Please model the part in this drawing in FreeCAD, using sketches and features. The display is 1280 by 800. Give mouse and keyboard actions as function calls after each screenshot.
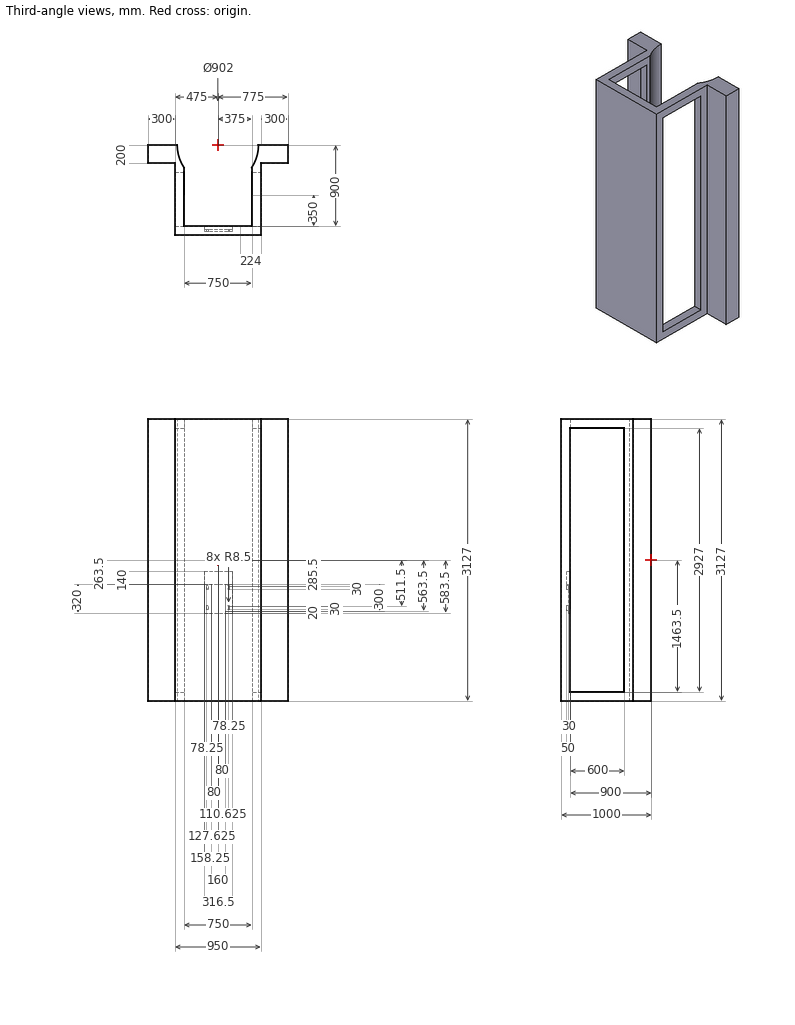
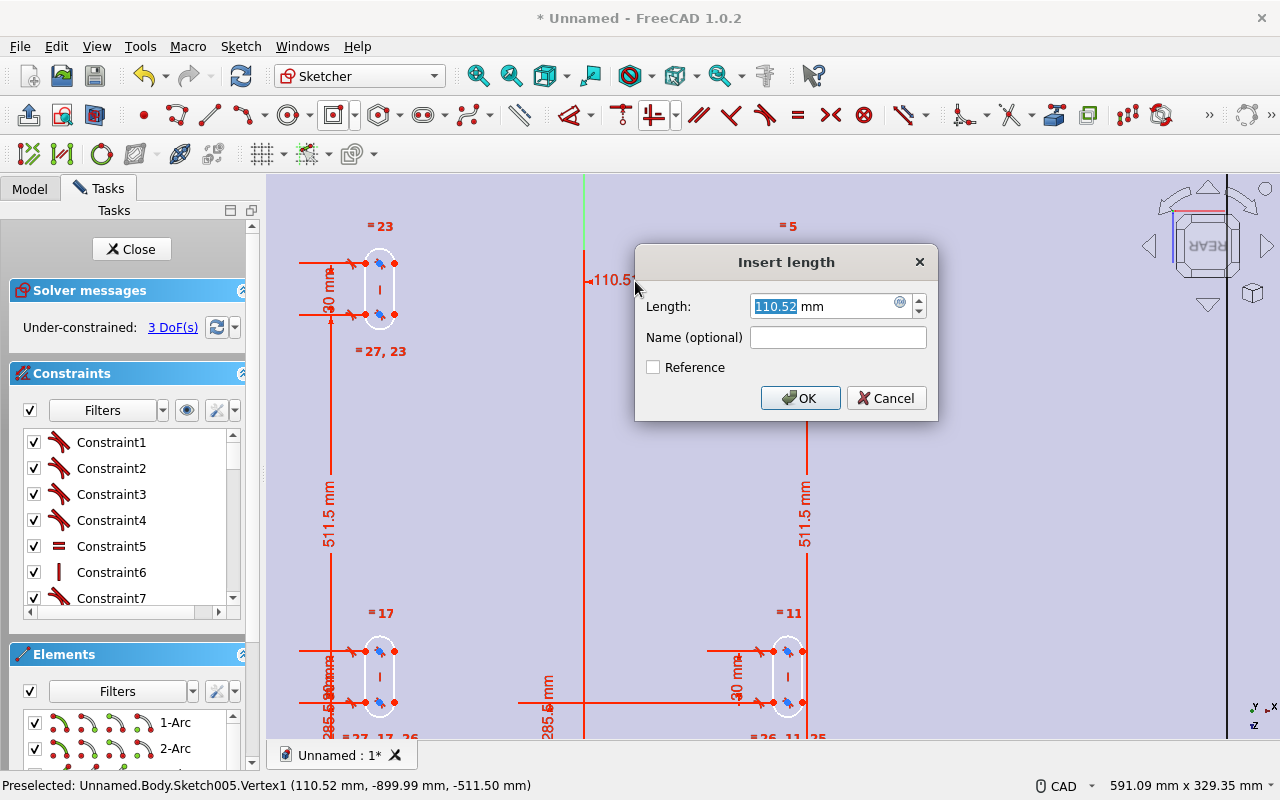
text(110.625)
key(Return)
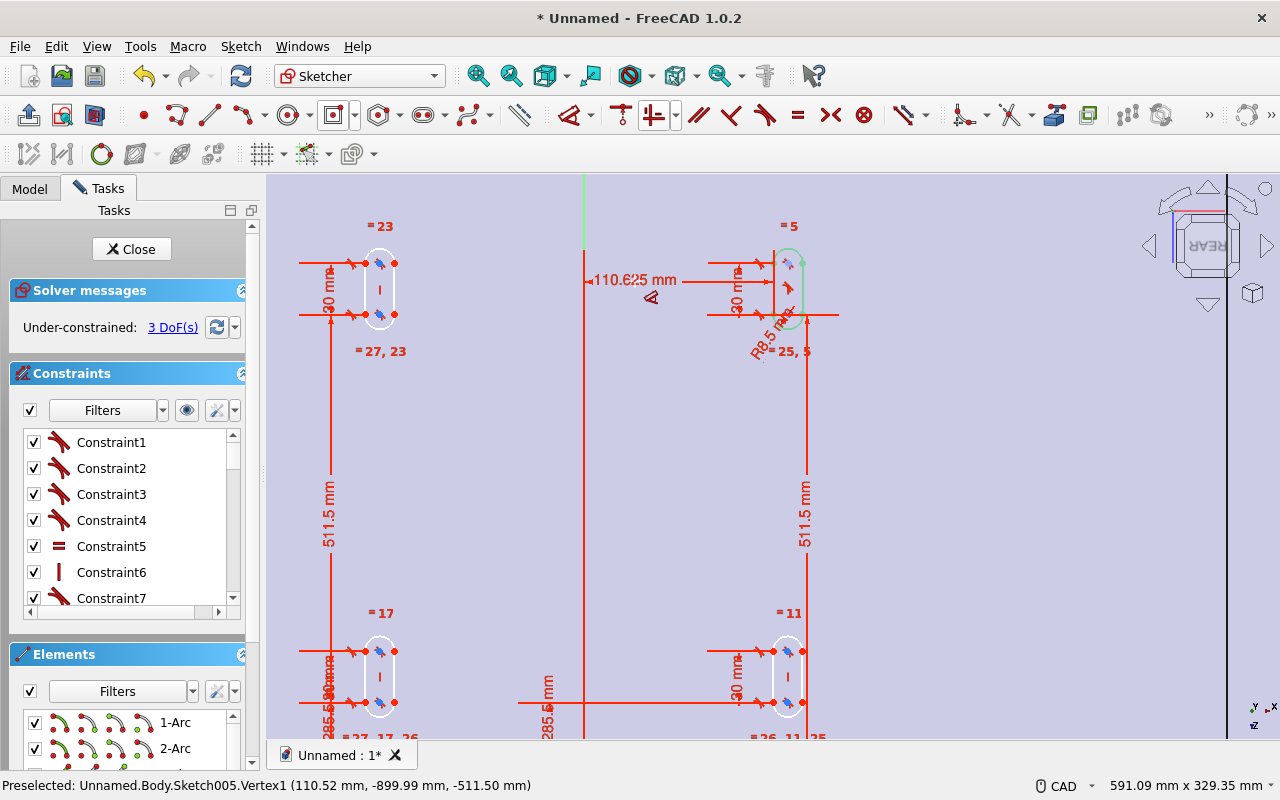
click(773, 703)
click(635, 669)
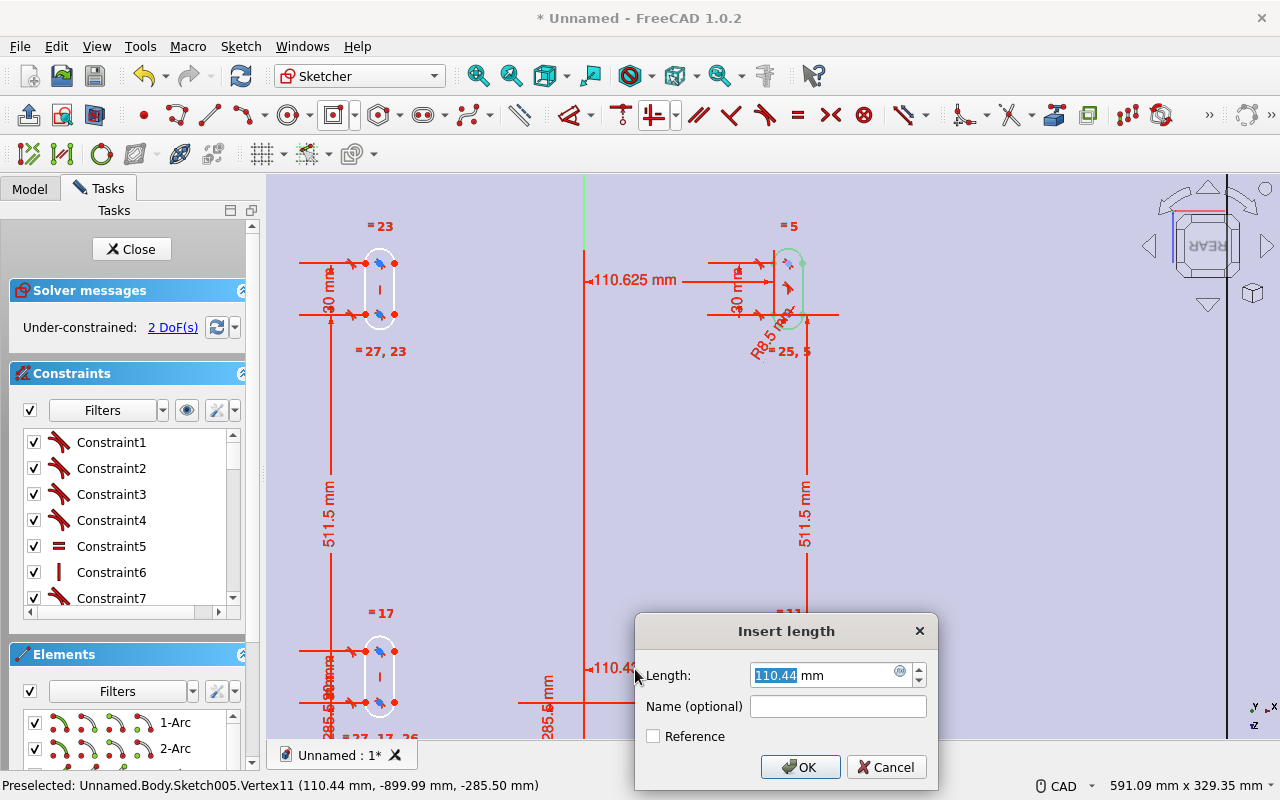
text(110.625)
key(Return)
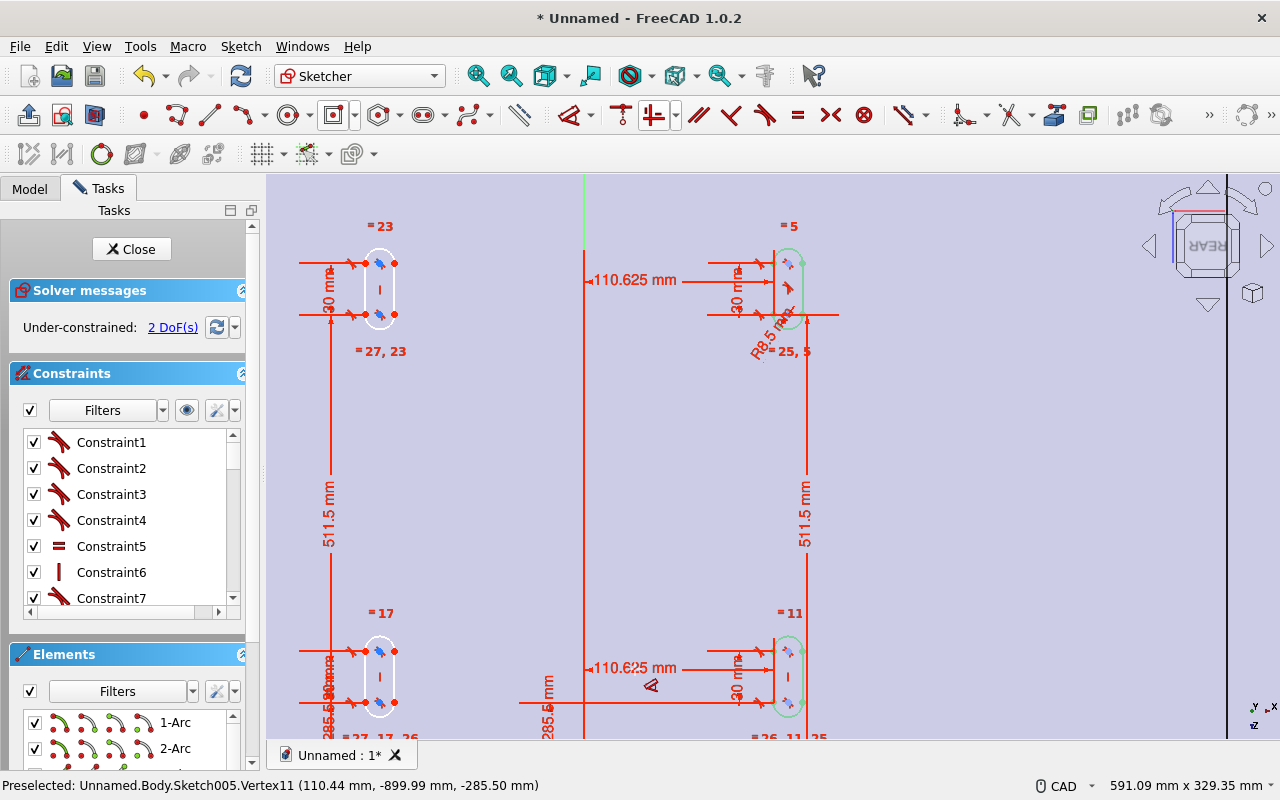
click(365, 703)
click(474, 669)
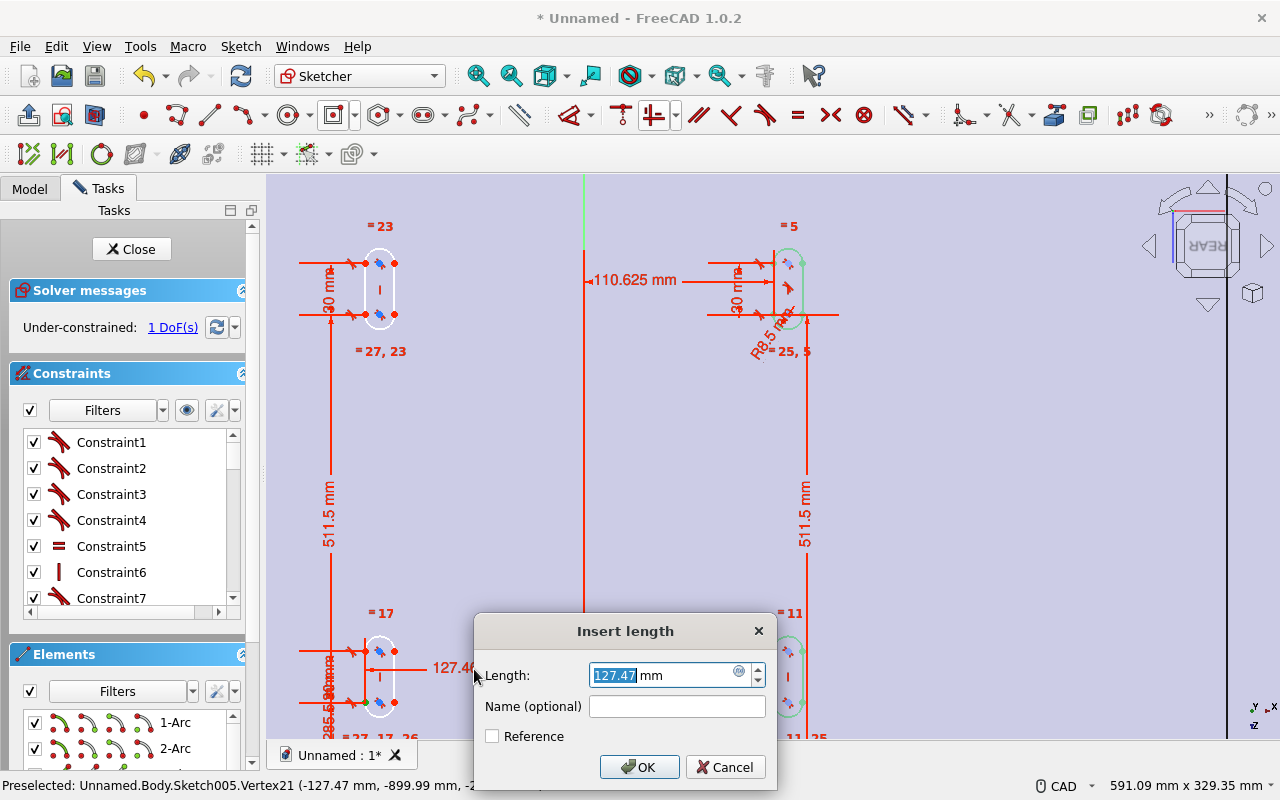
text(127.625)
key(Return)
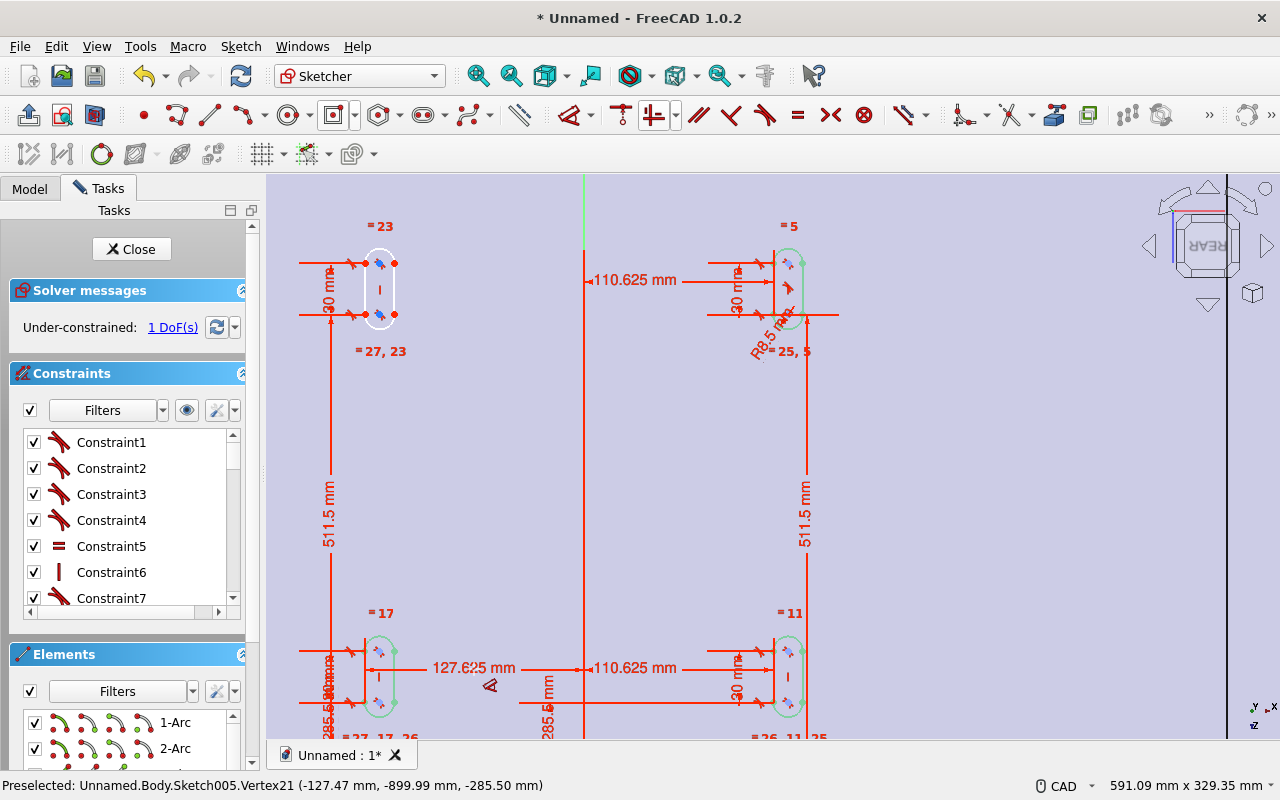
click(365, 315)
click(475, 281)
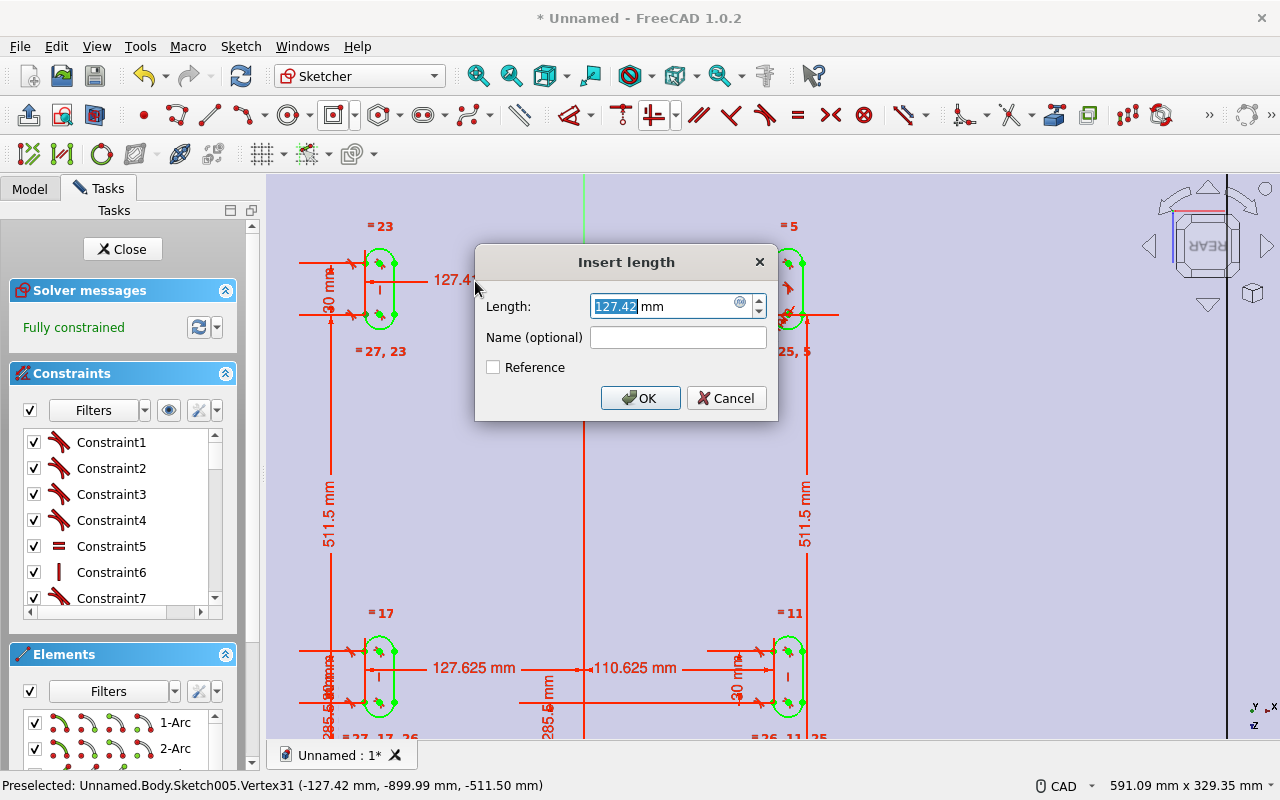
text(127.625)
key(Return)
key(Escape)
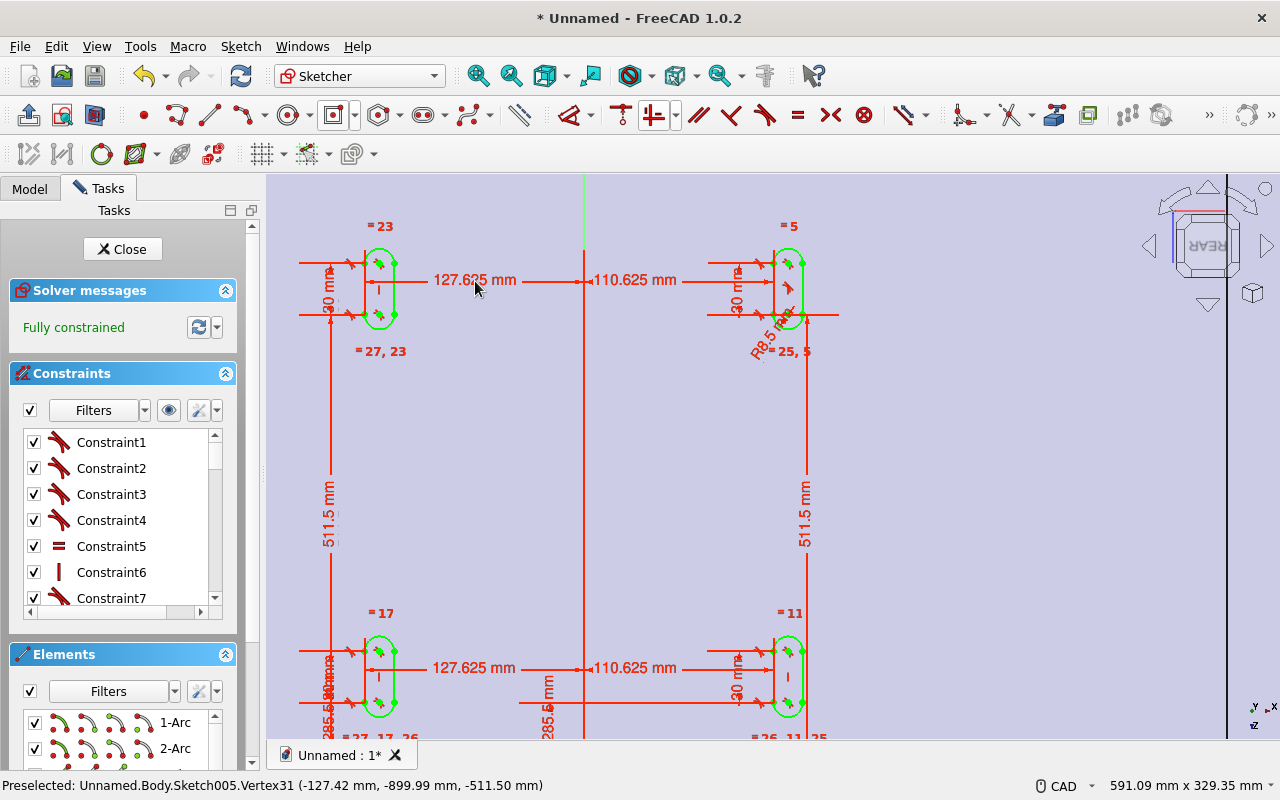
click(123, 249)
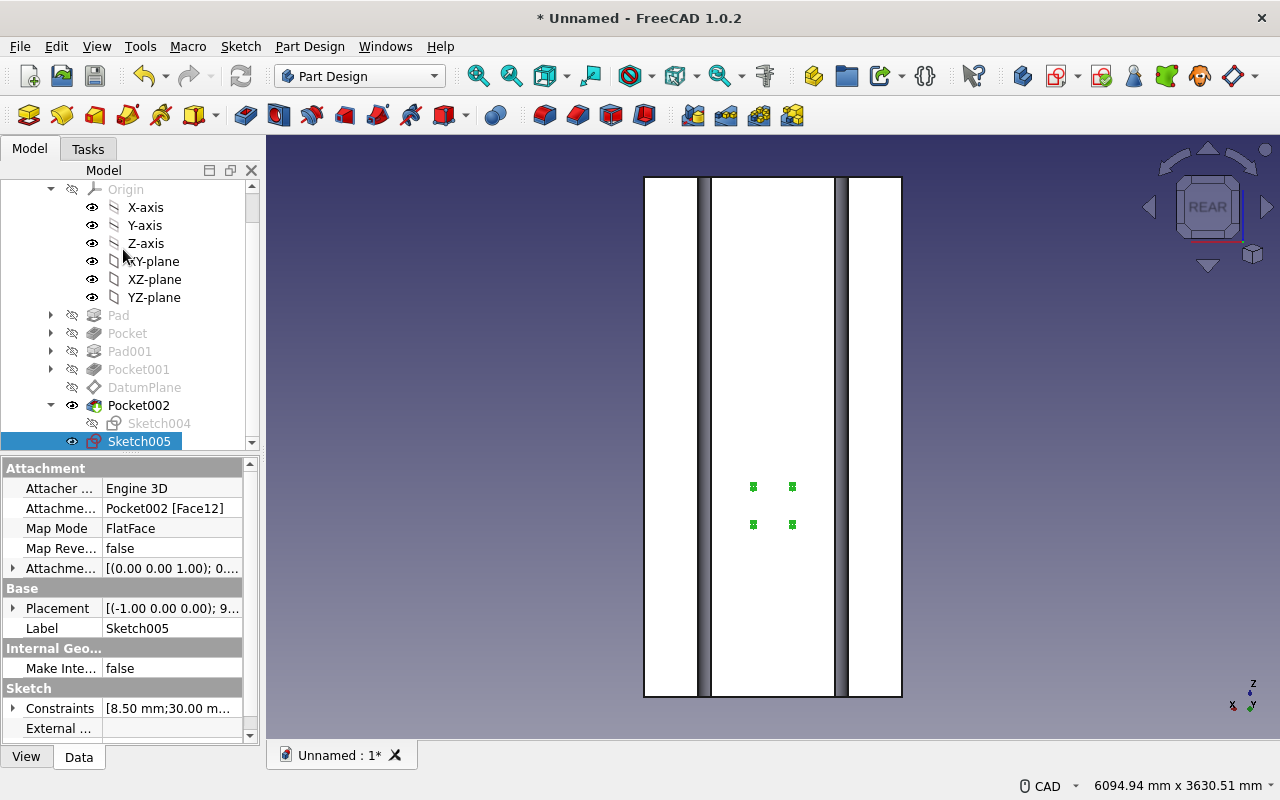
click(246, 116)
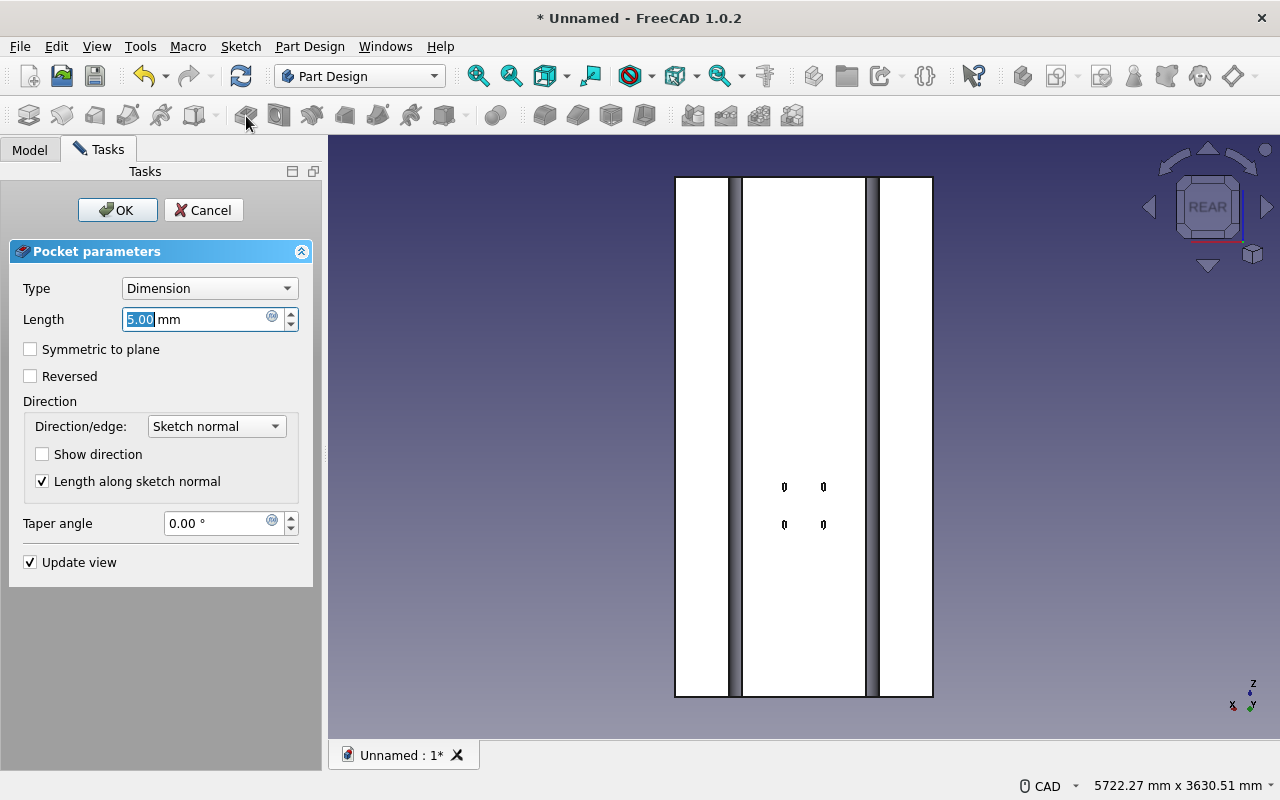
text(50)
key(Tab)